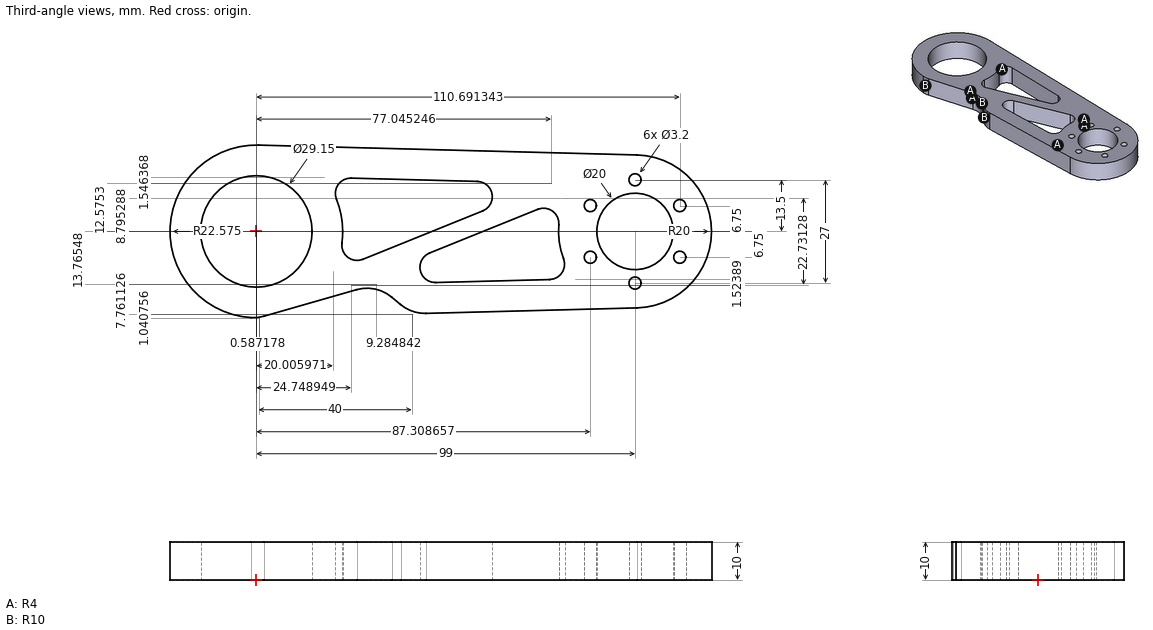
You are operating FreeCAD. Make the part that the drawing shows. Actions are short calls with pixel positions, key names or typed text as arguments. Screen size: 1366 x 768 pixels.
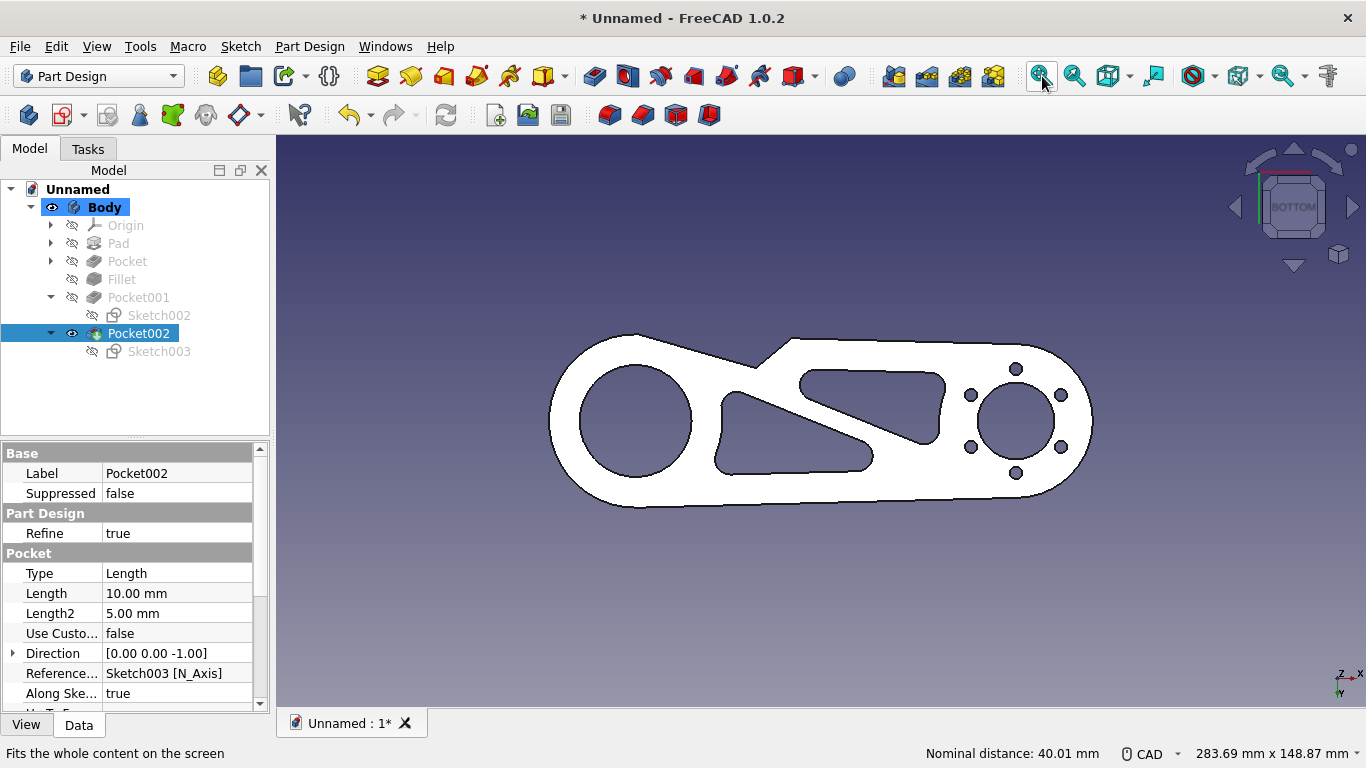
key(4)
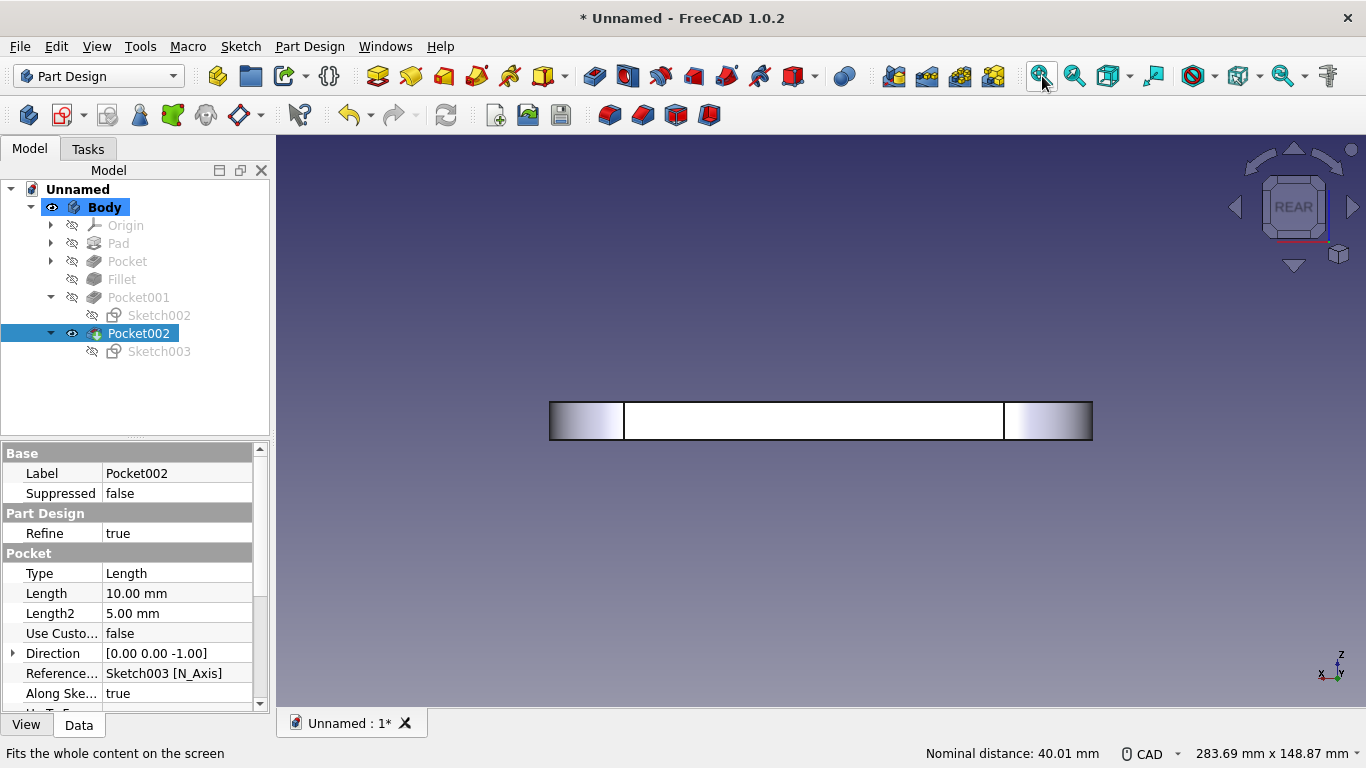
key(6)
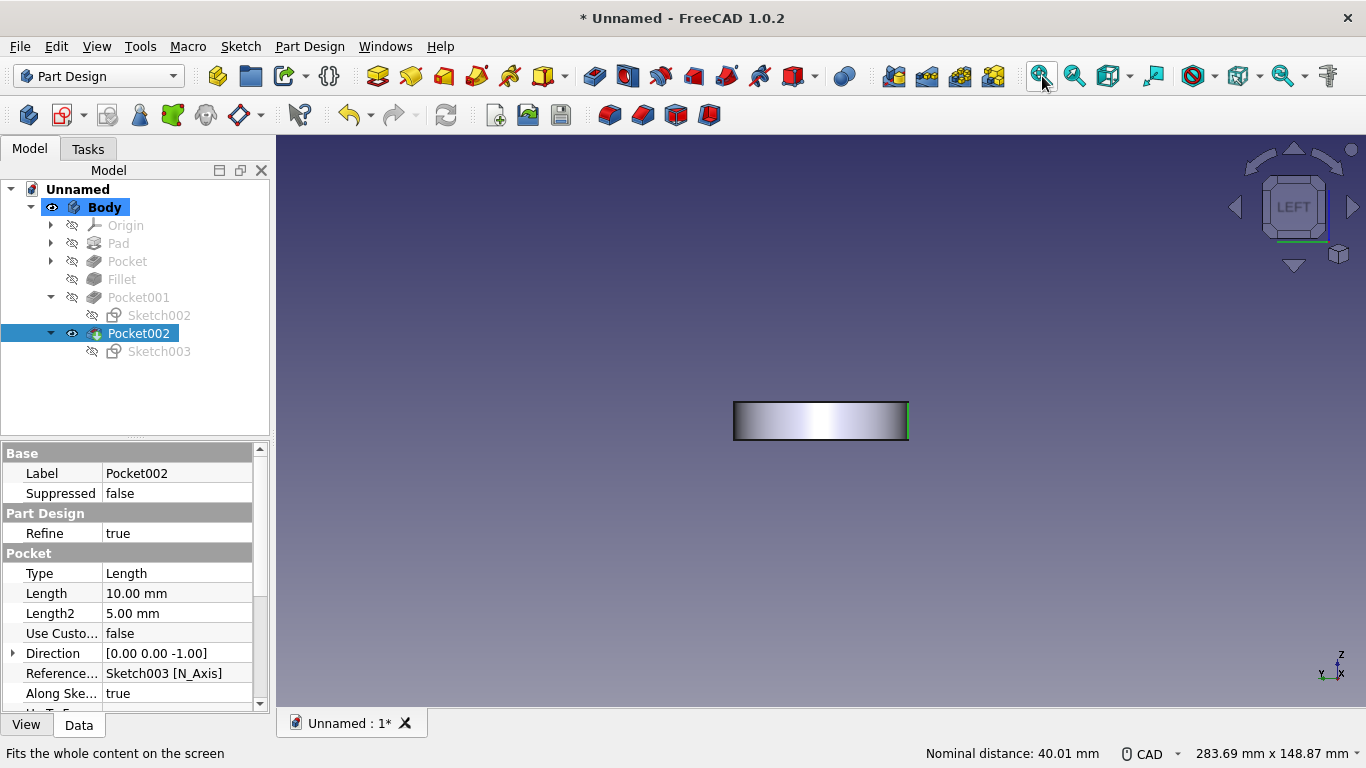
click(1042, 76)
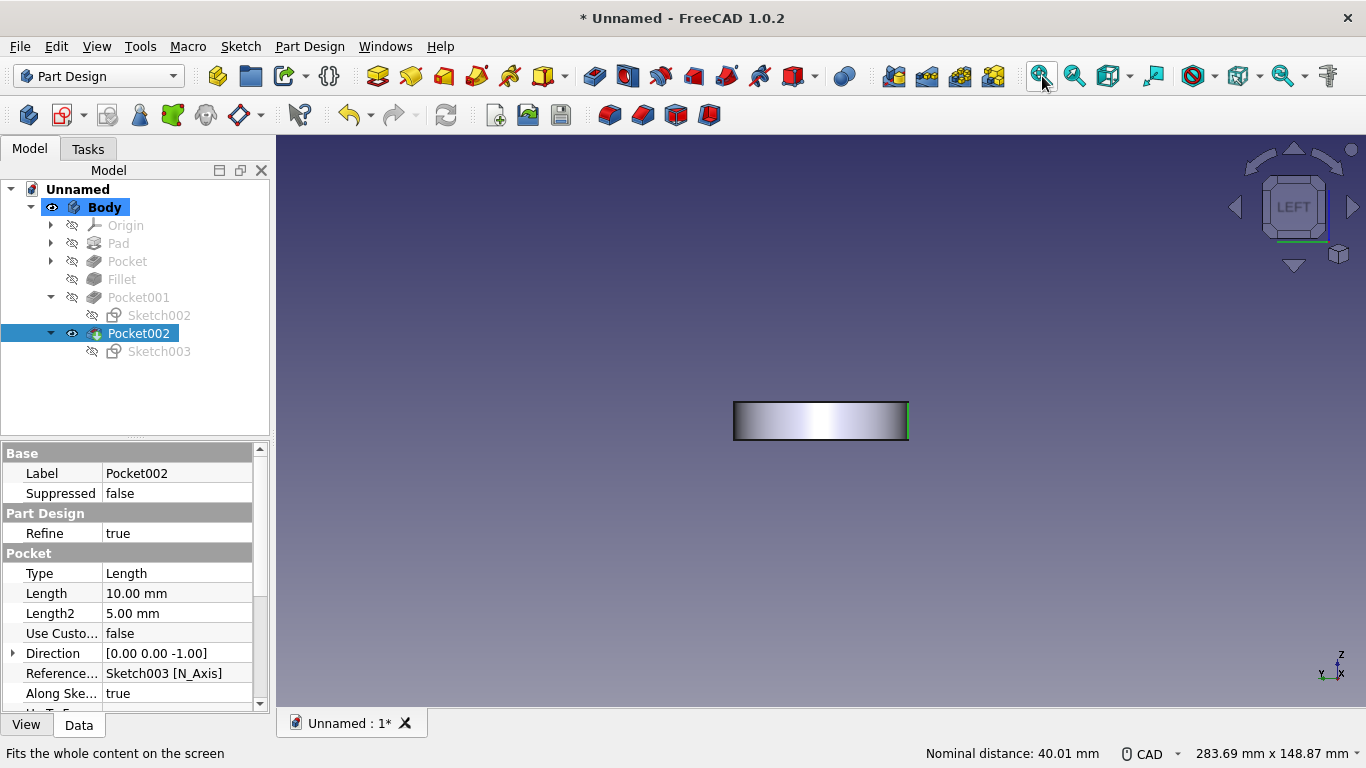
key(v)
key(3)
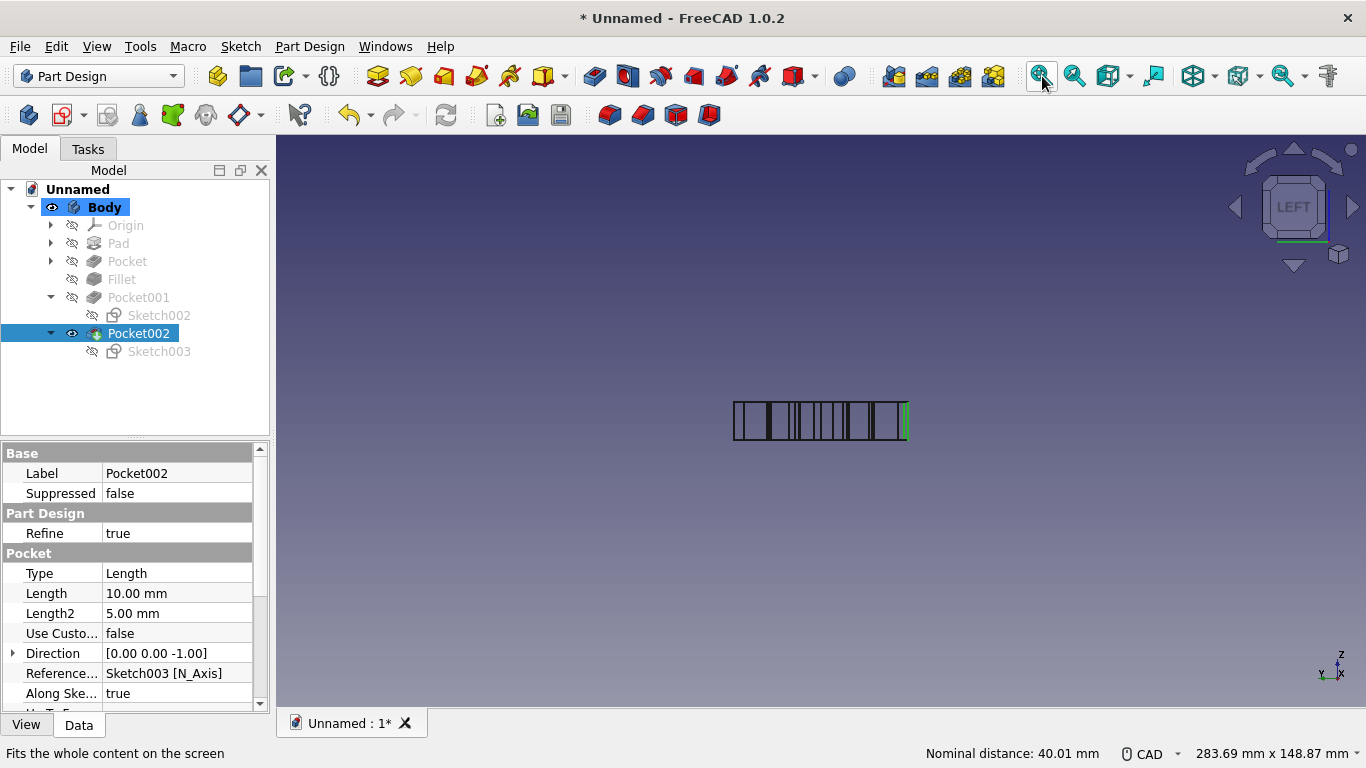
key(0)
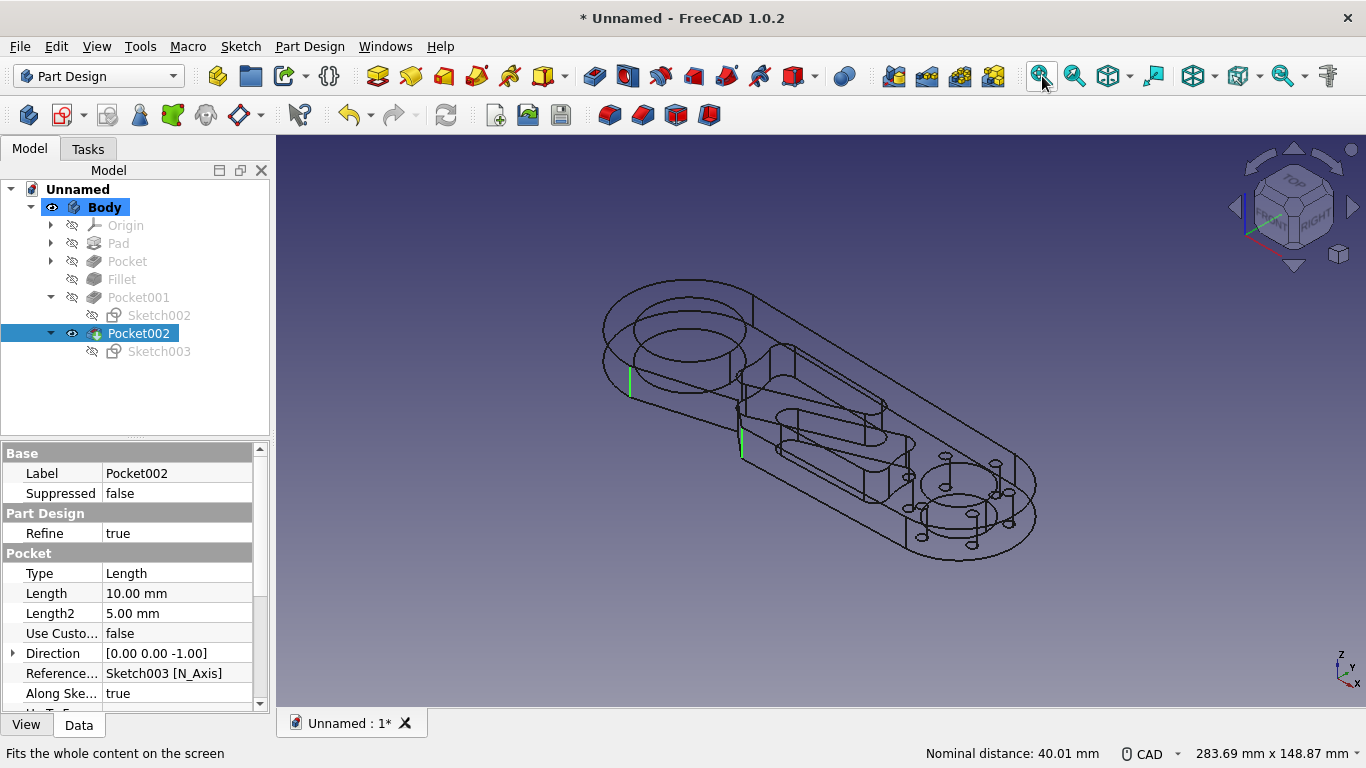
scroll(738, 415, up, 6)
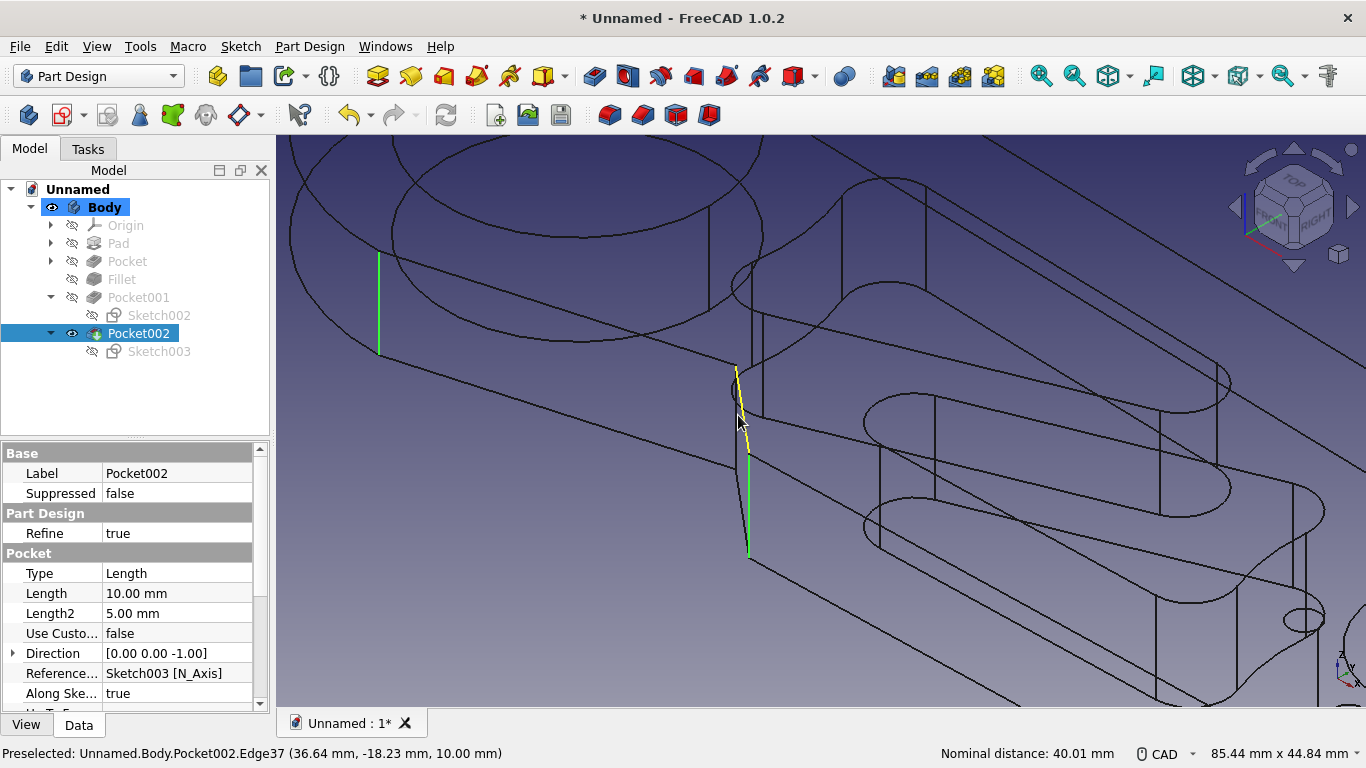
click(736, 416, ctrl)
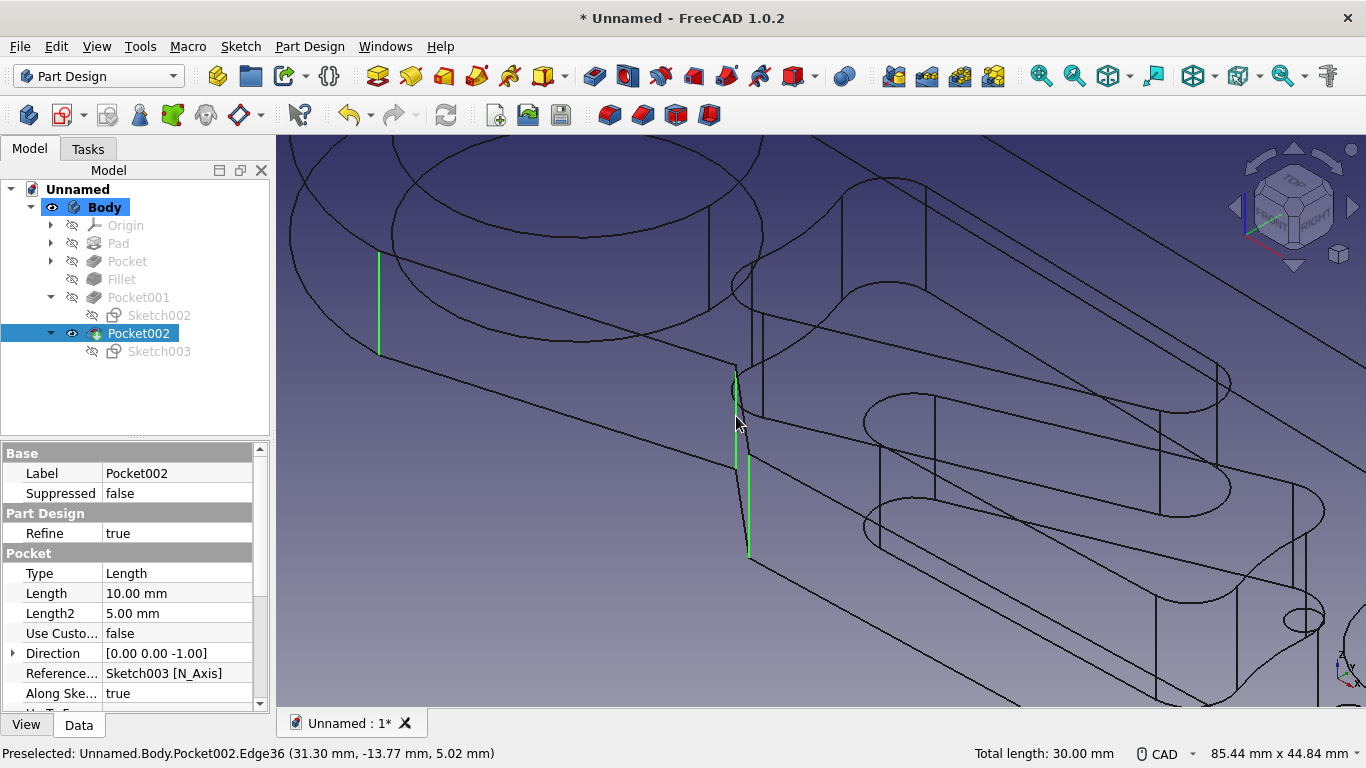
key(v)
key(1)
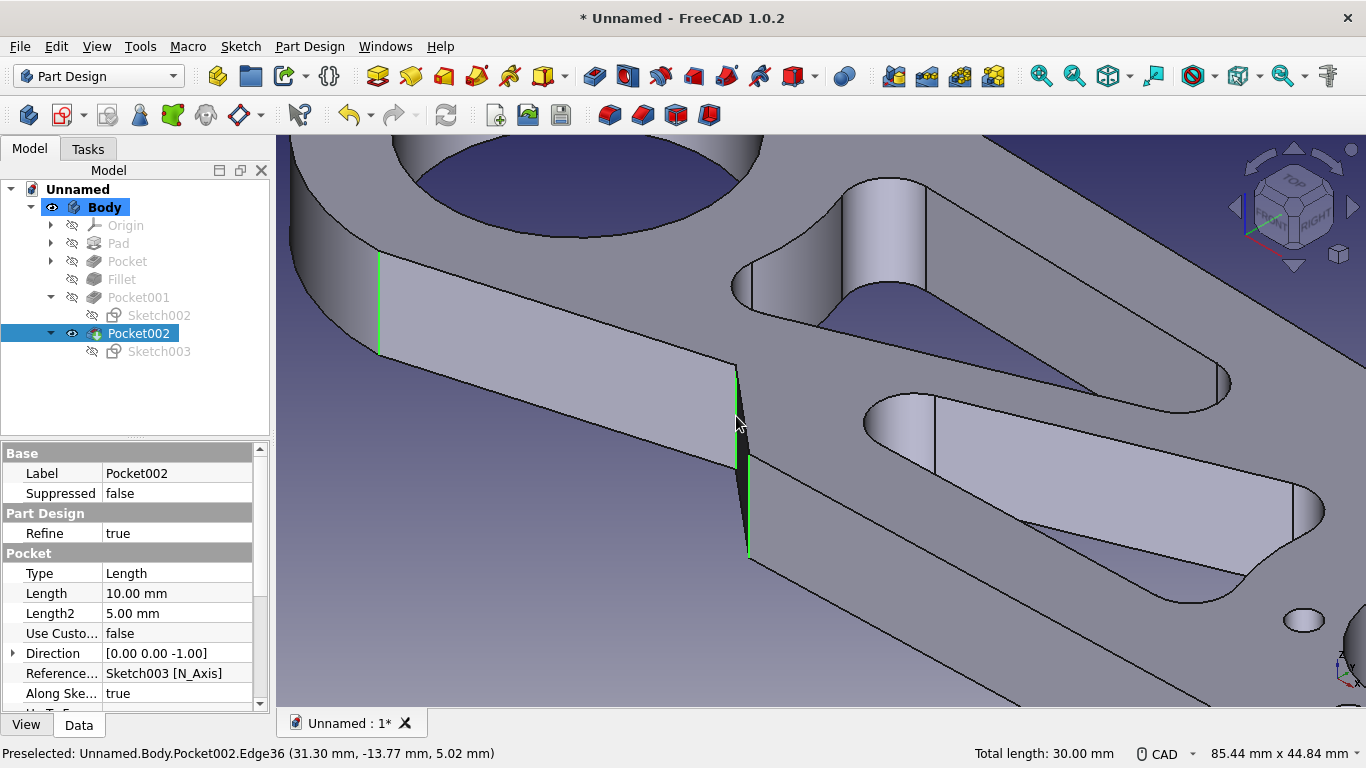
click(610, 116)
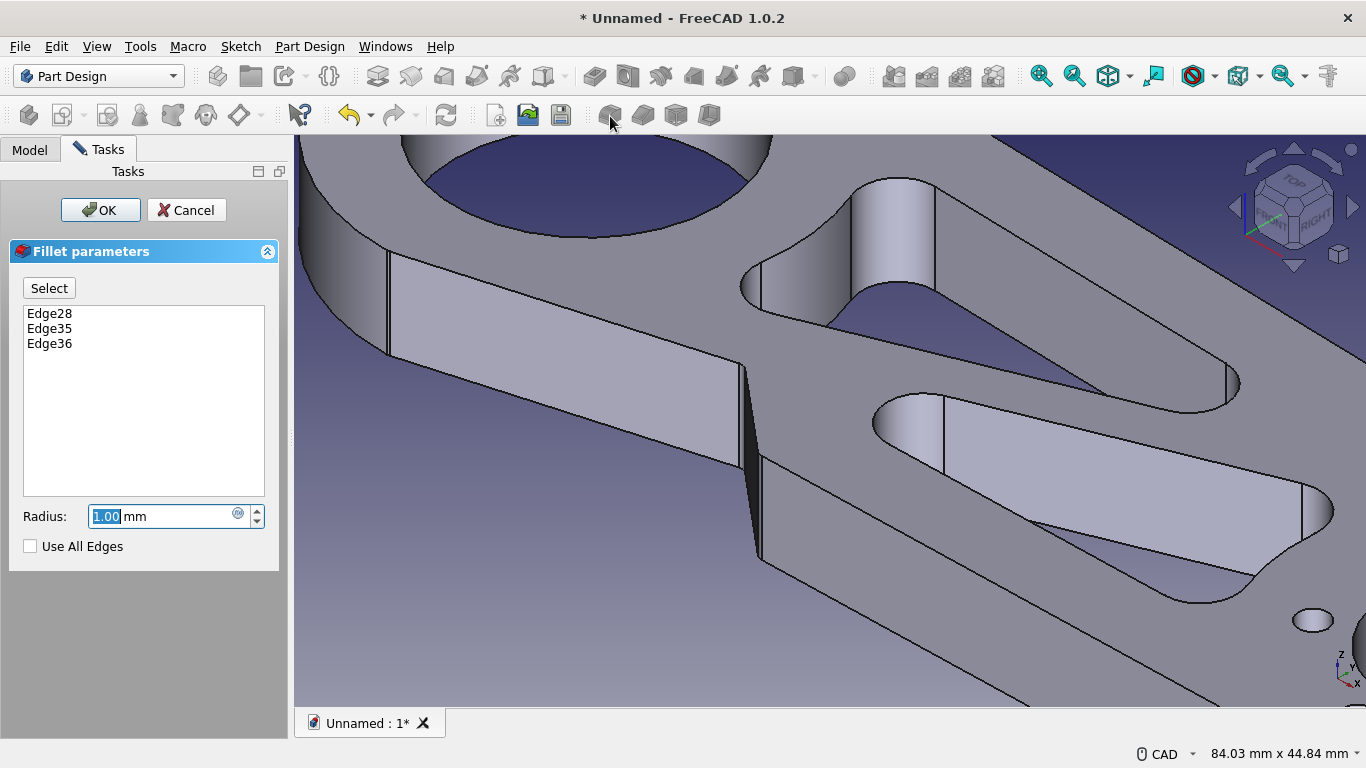
text(10)
key(Tab)